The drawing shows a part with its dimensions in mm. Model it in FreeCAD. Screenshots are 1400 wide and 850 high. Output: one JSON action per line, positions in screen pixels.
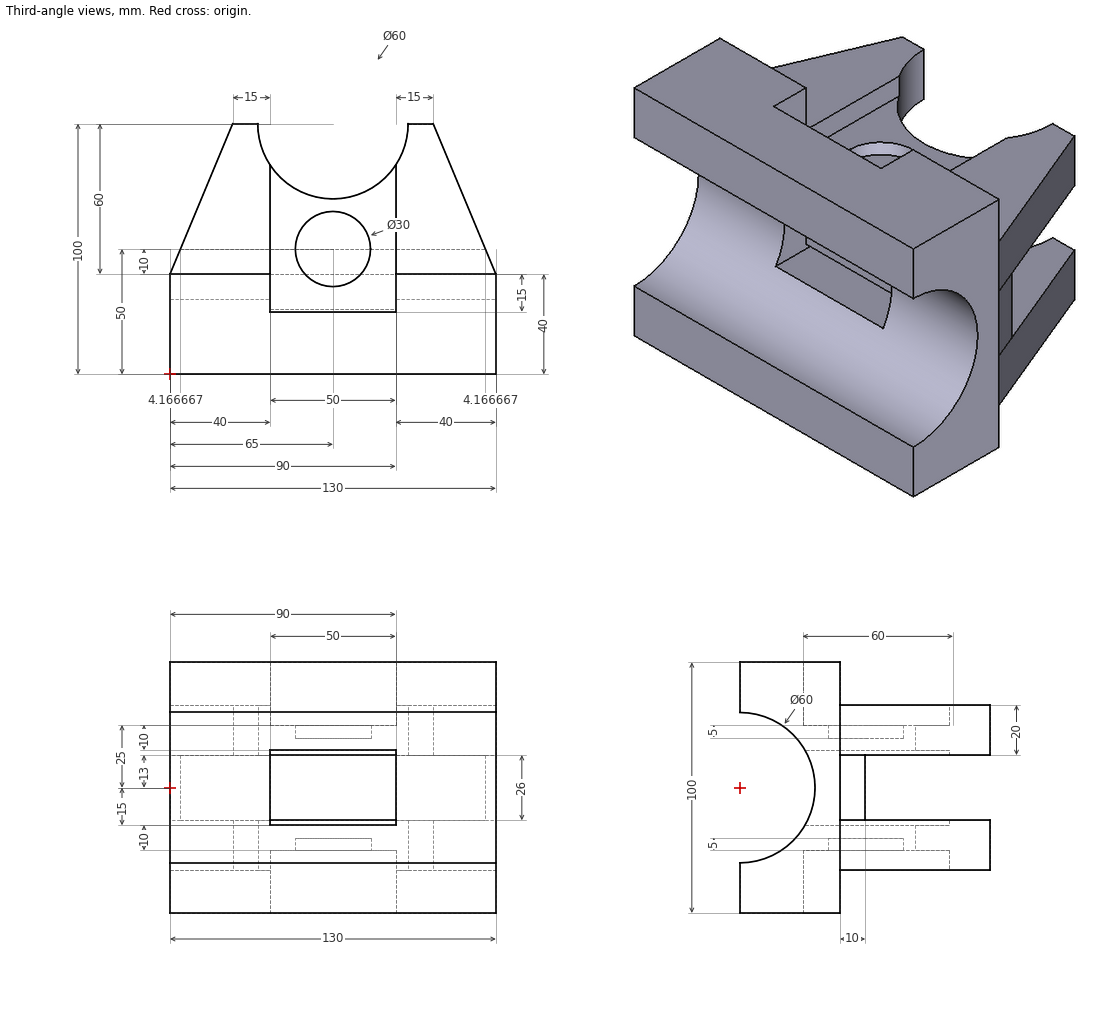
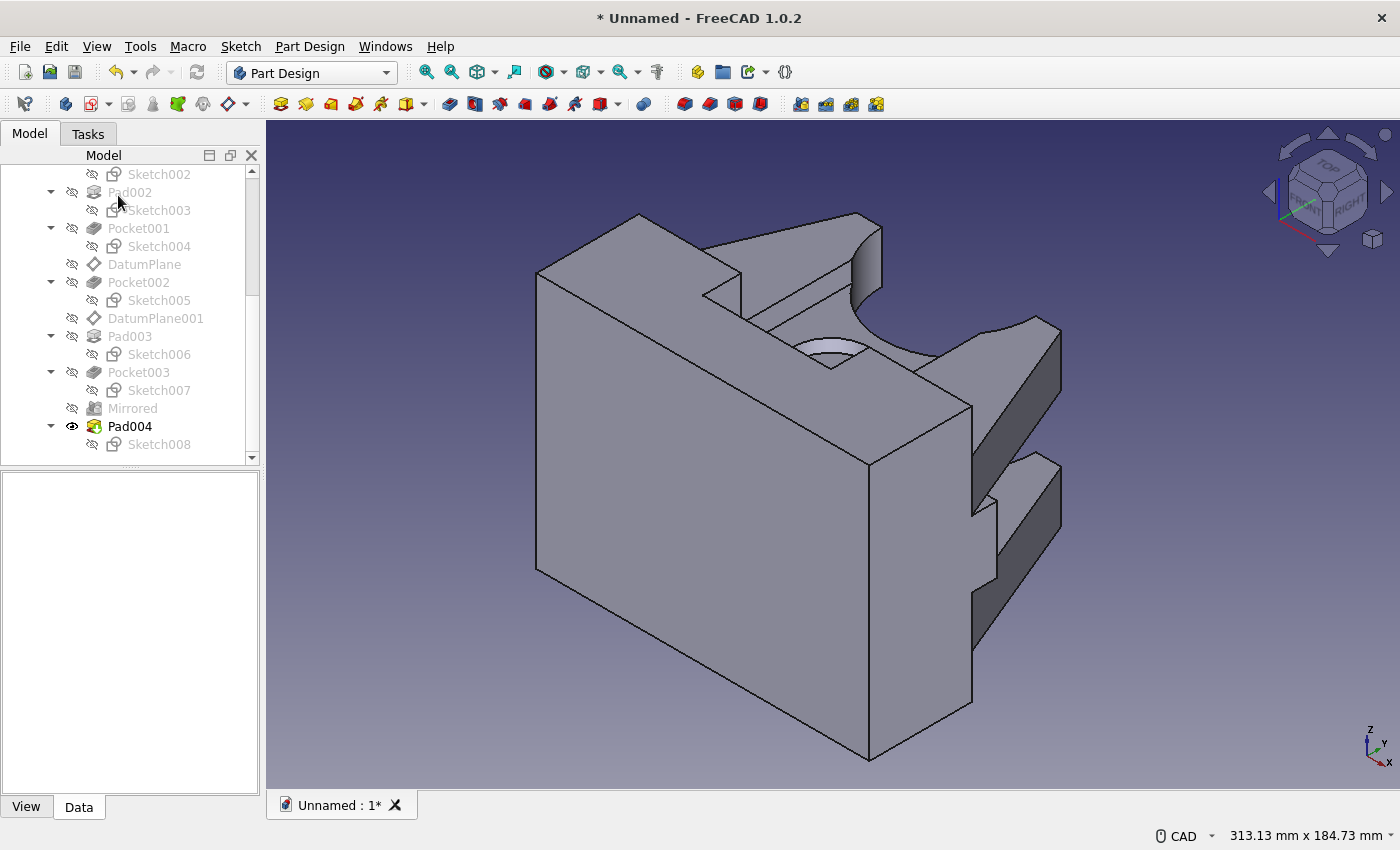
{"action": "scroll", "coordinate": [988, 501], "scroll_direction": "up", "scroll_amount": 5}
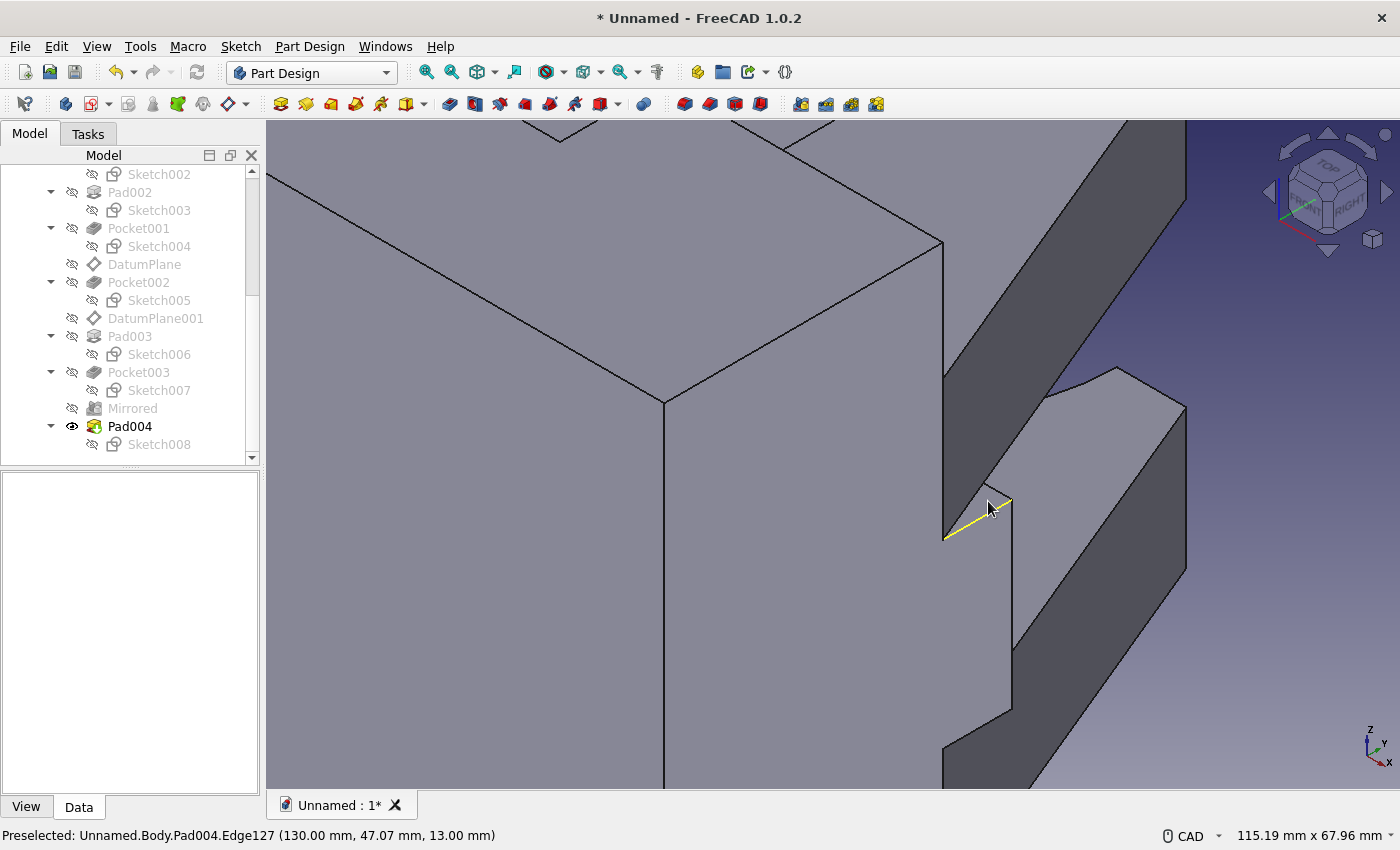
{"action": "left_click", "coordinate": [987, 501]}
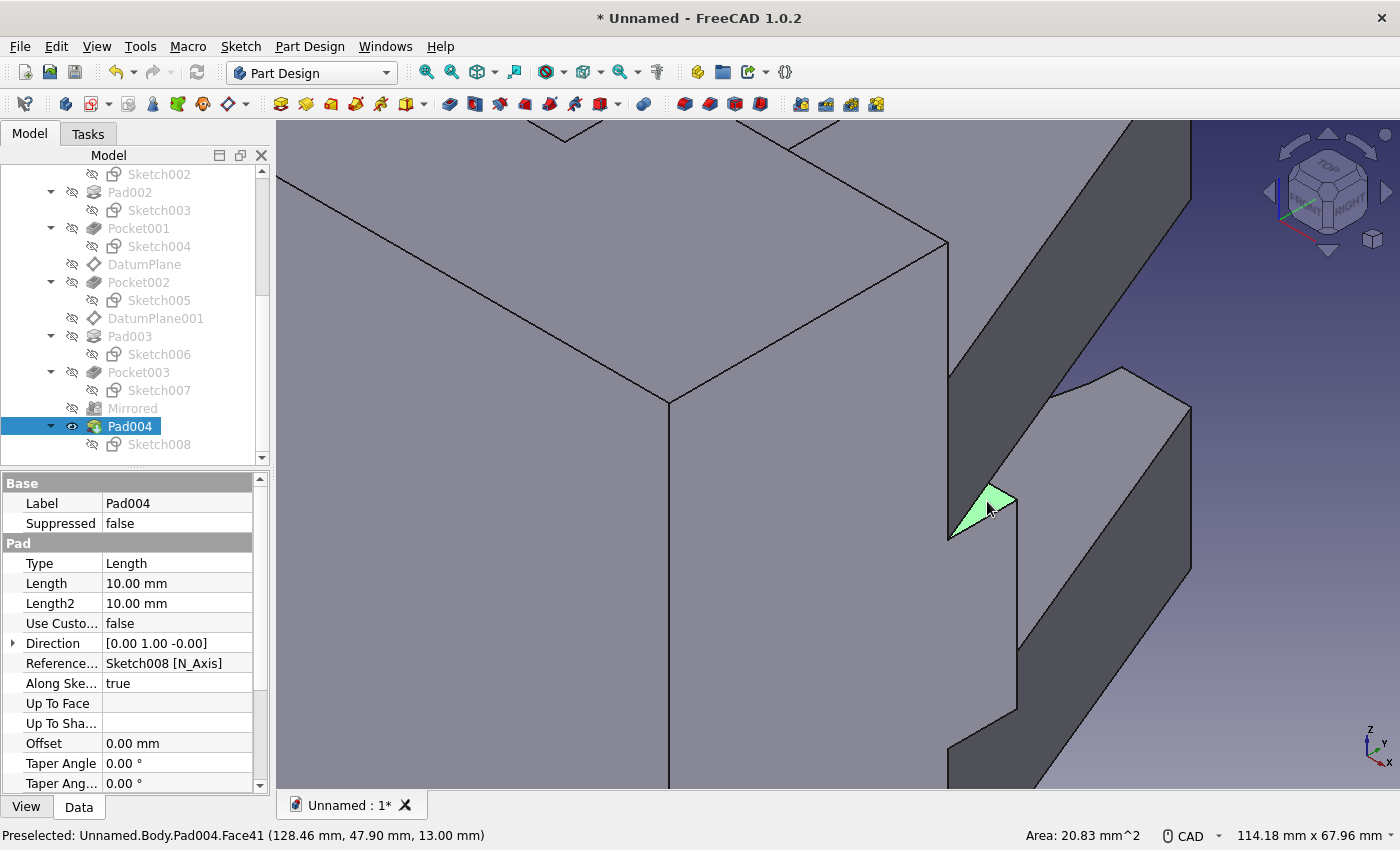
{"action": "left_click", "coordinate": [90, 104]}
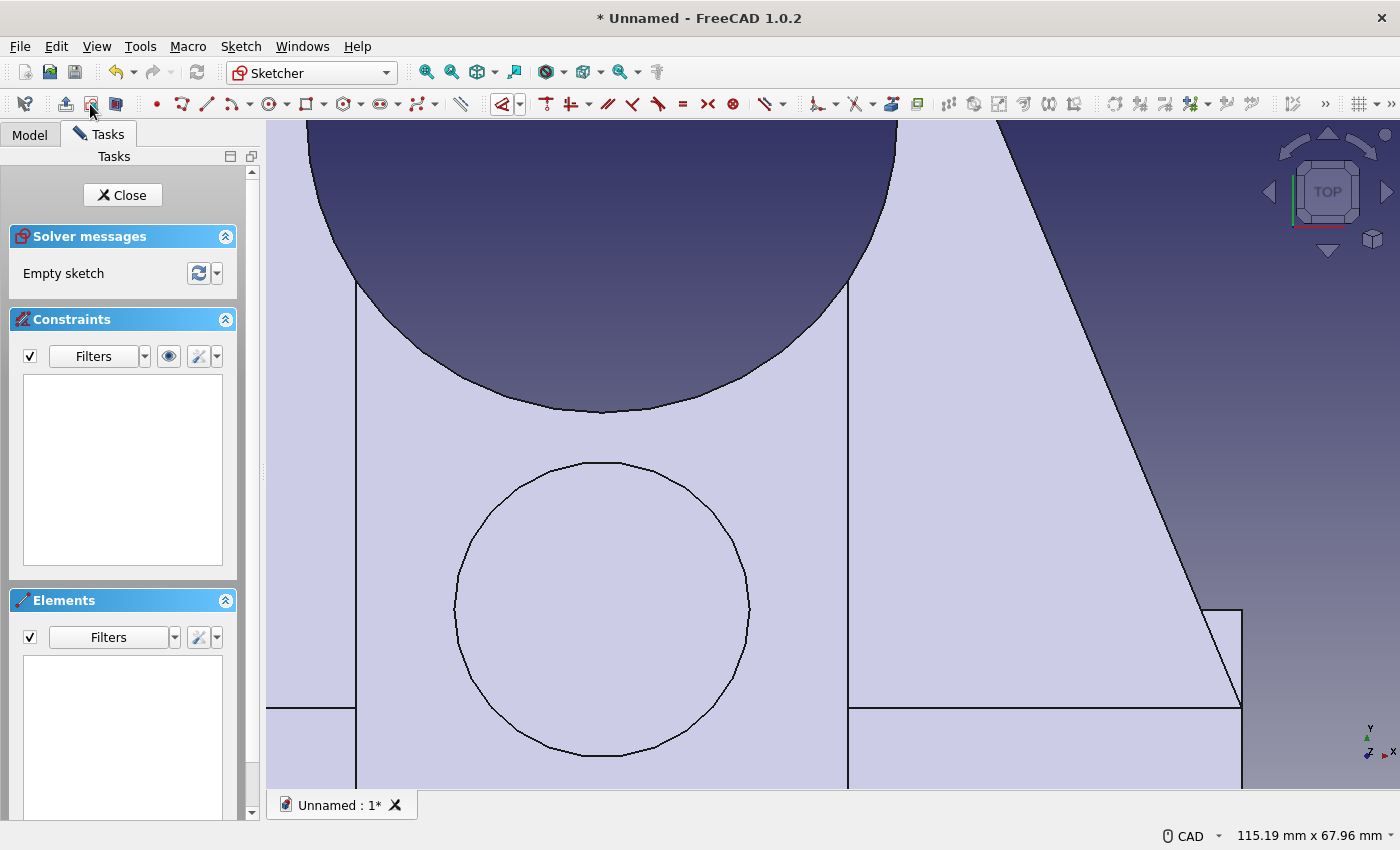
{"action": "left_click", "coordinate": [116, 104]}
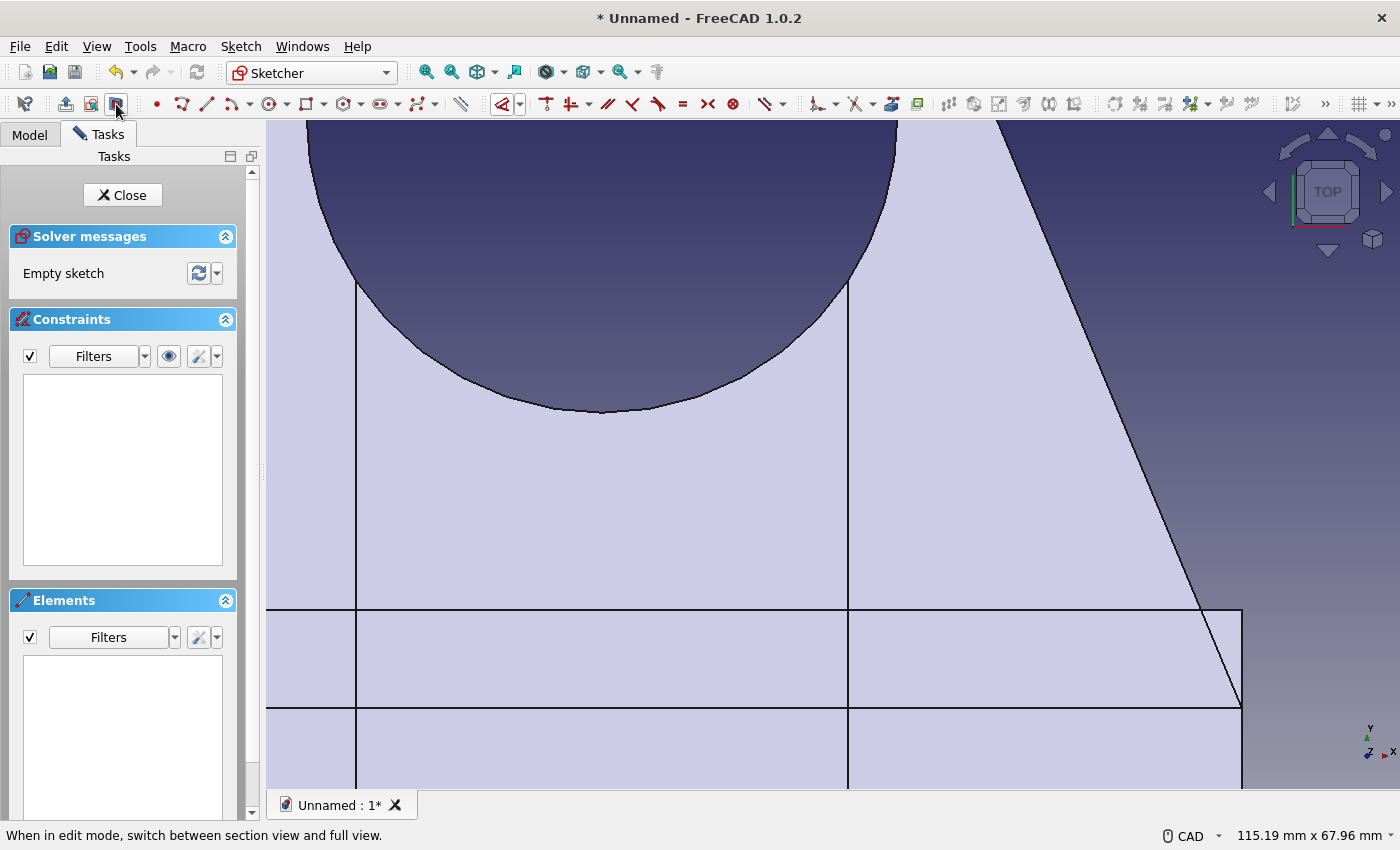
{"action": "scroll", "coordinate": [764, 454], "scroll_direction": "down", "scroll_amount": 5}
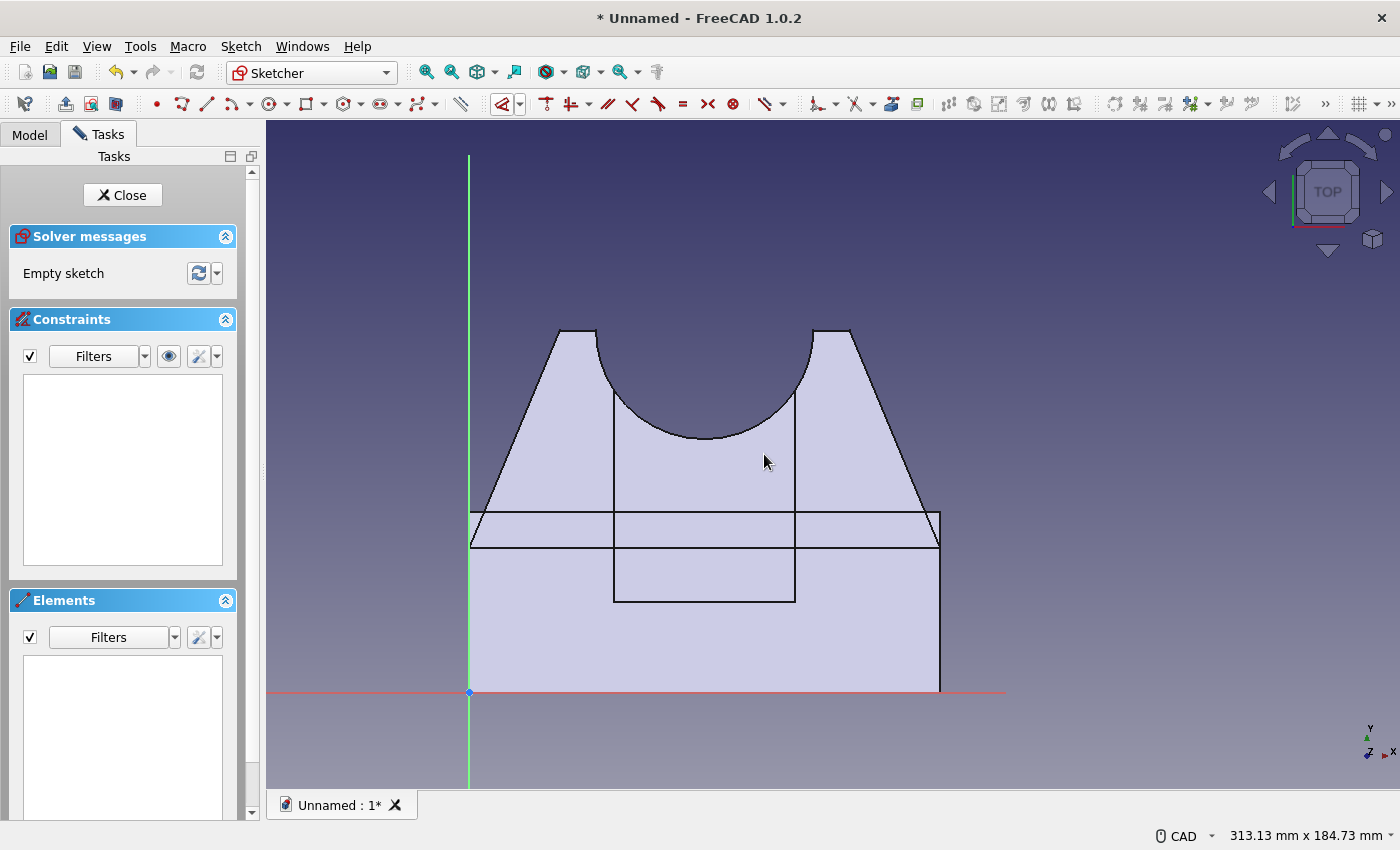
{"action": "scroll", "coordinate": [448, 537], "scroll_direction": "up", "scroll_amount": 12}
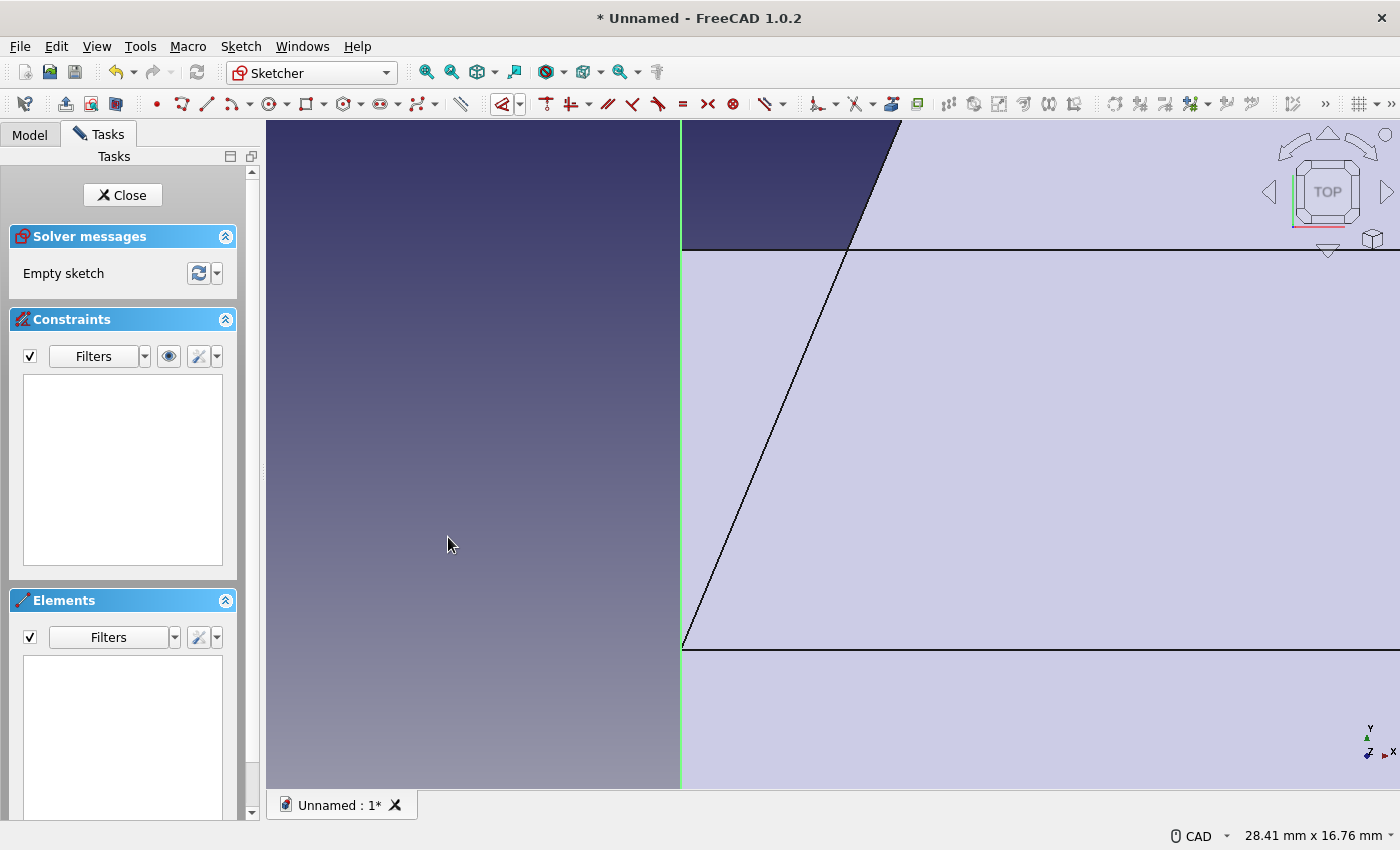
{"action": "left_click", "coordinate": [182, 104]}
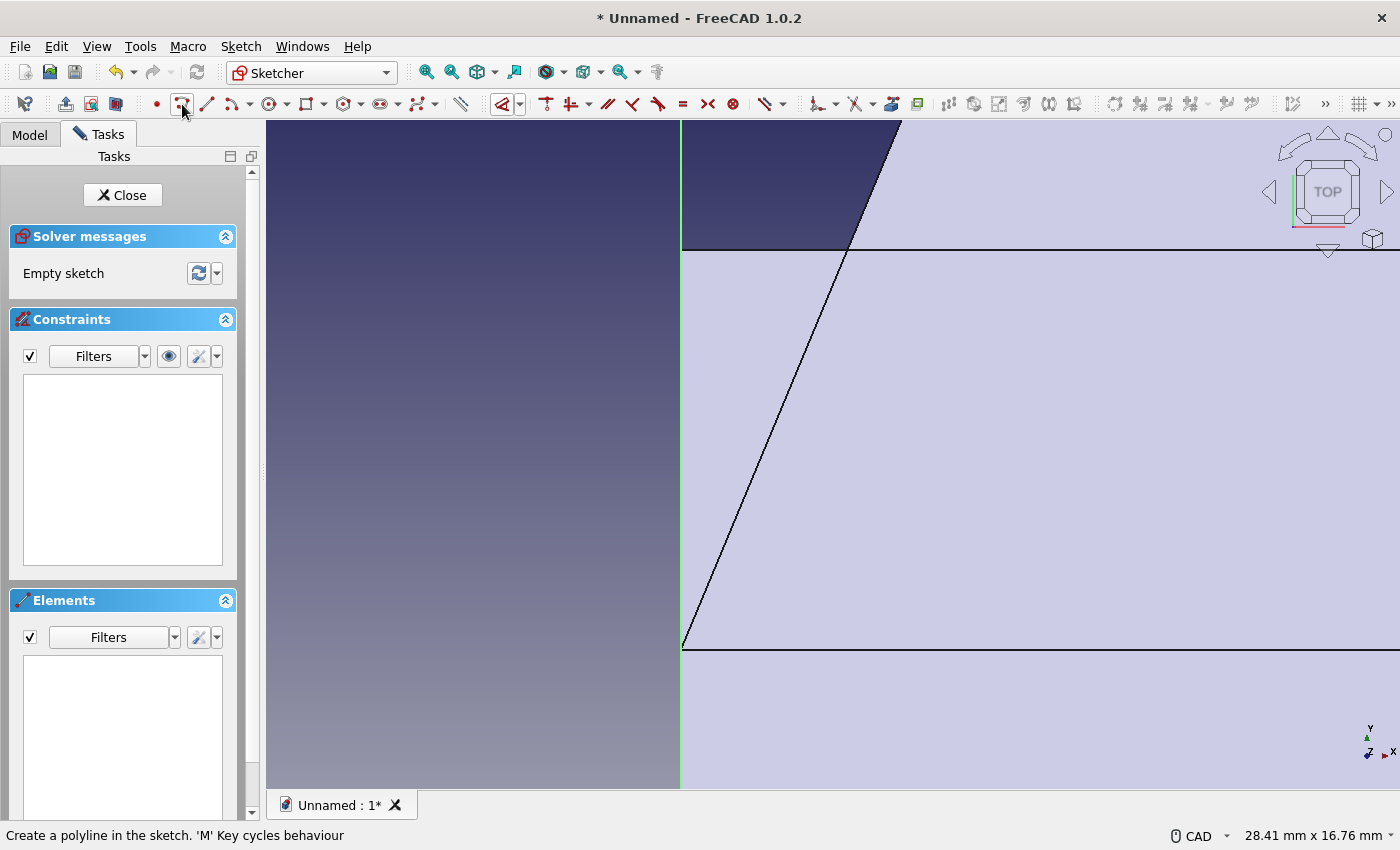
{"action": "left_click", "coordinate": [681, 650]}
{"action": "left_click", "coordinate": [847, 250]}
{"action": "left_click", "coordinate": [690, 250]}
{"action": "left_click", "coordinate": [681, 651]}
{"action": "key", "text": "Escape"}
{"action": "key", "text": "Escape"}